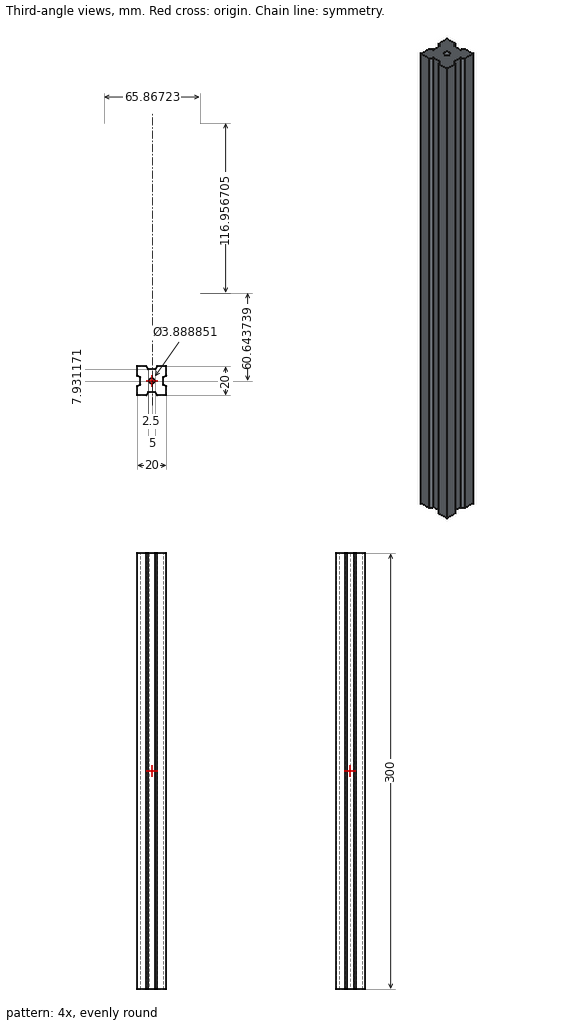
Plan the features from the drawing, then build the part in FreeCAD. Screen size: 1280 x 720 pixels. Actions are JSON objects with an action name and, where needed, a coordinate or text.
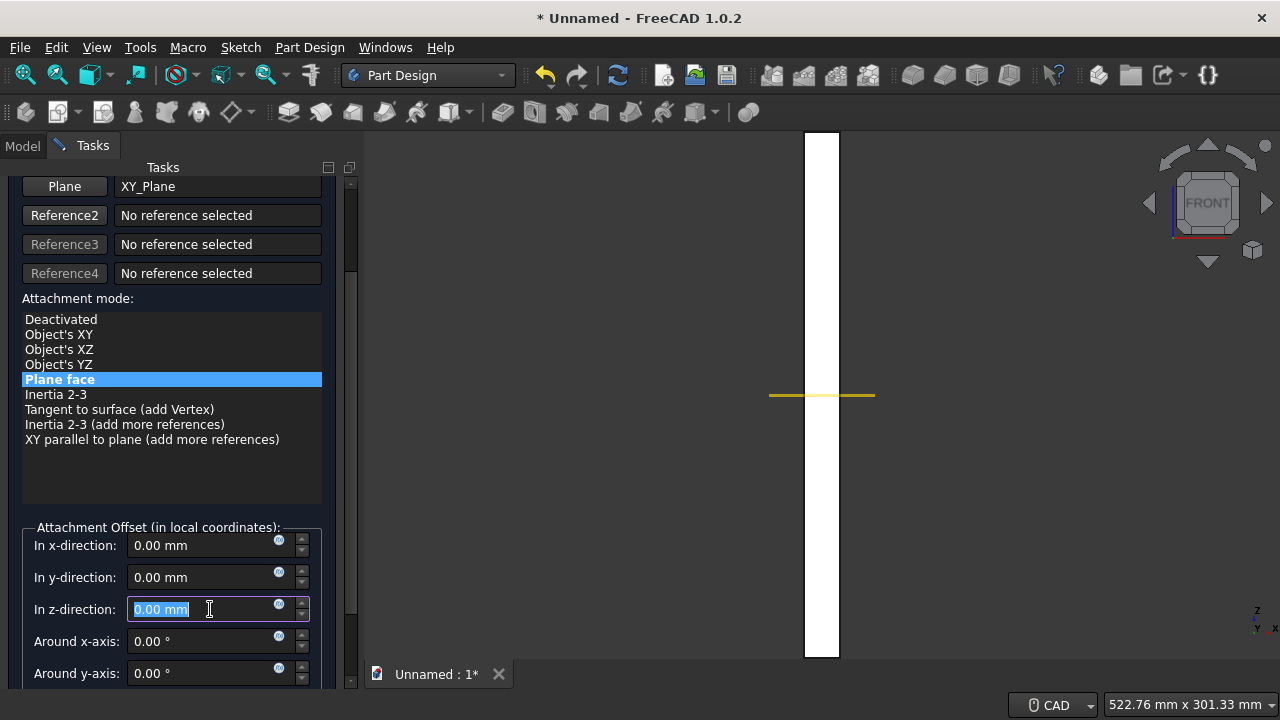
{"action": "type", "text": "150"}
{"action": "key", "text": "Tab"}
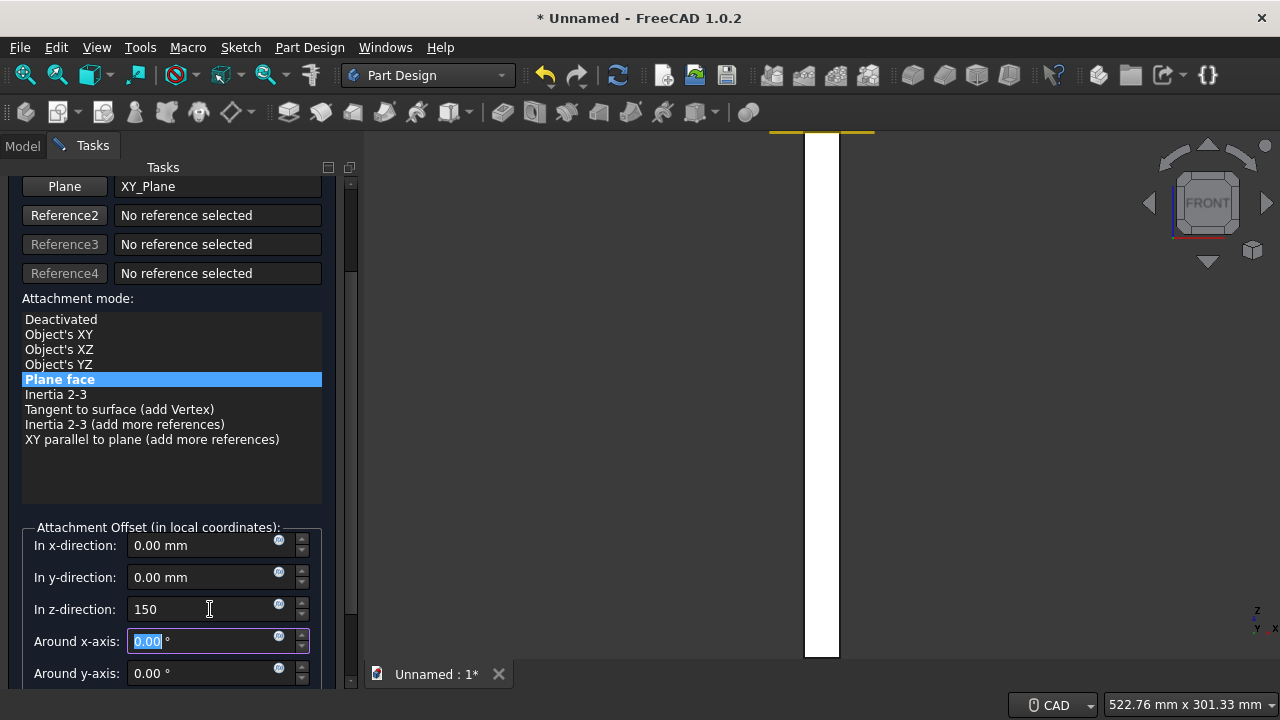
{"action": "scroll", "coordinate": [351, 432], "scroll_direction": "up", "scroll_amount": 3}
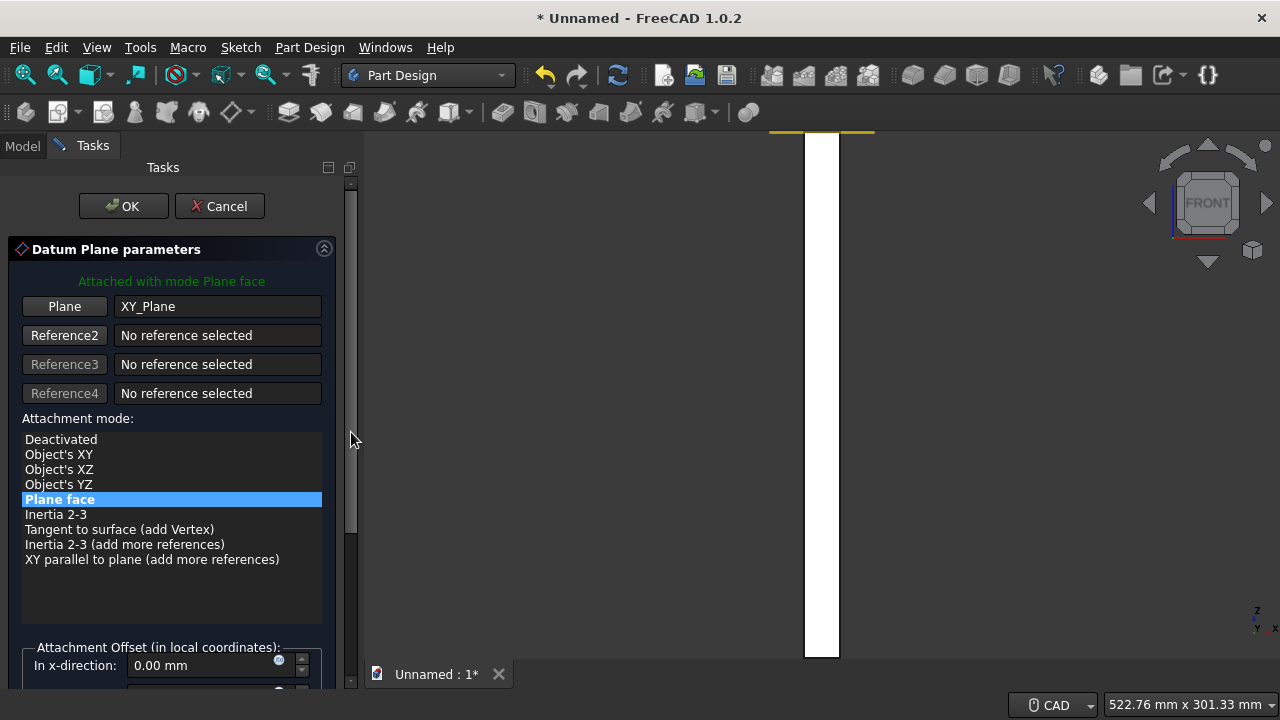
{"action": "left_click", "coordinate": [124, 206]}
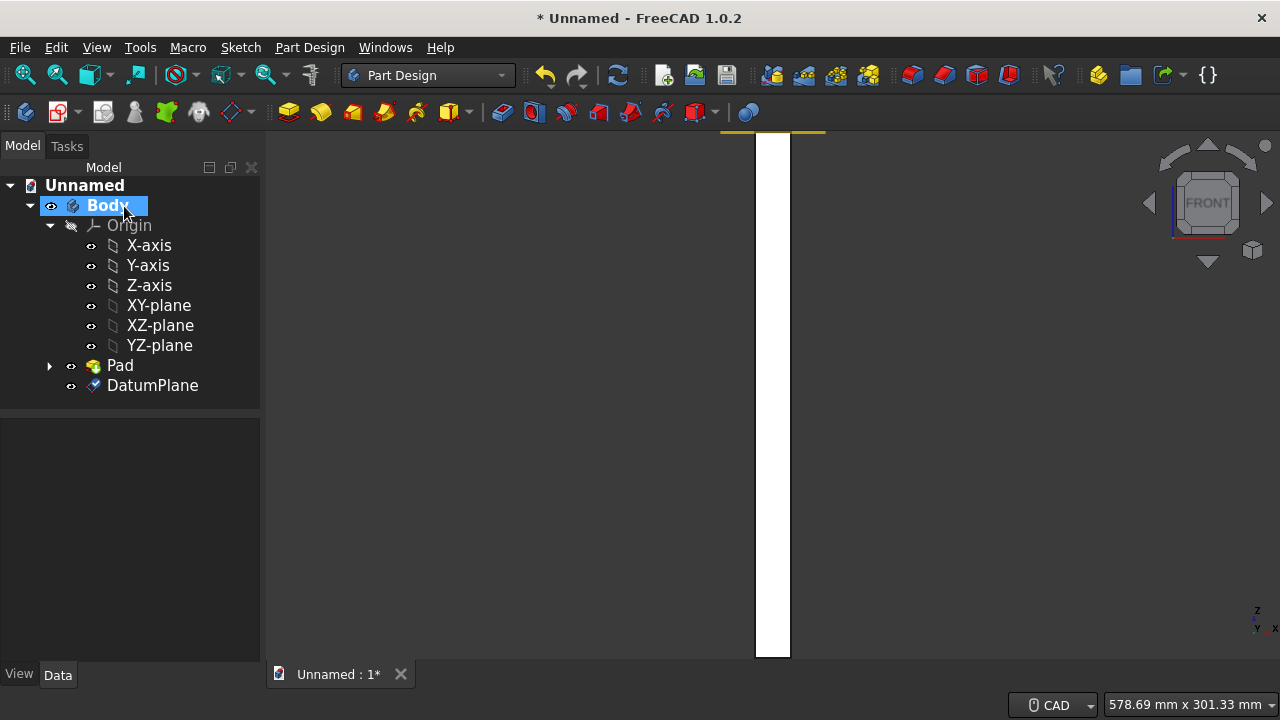
{"action": "left_click", "coordinate": [116, 386]}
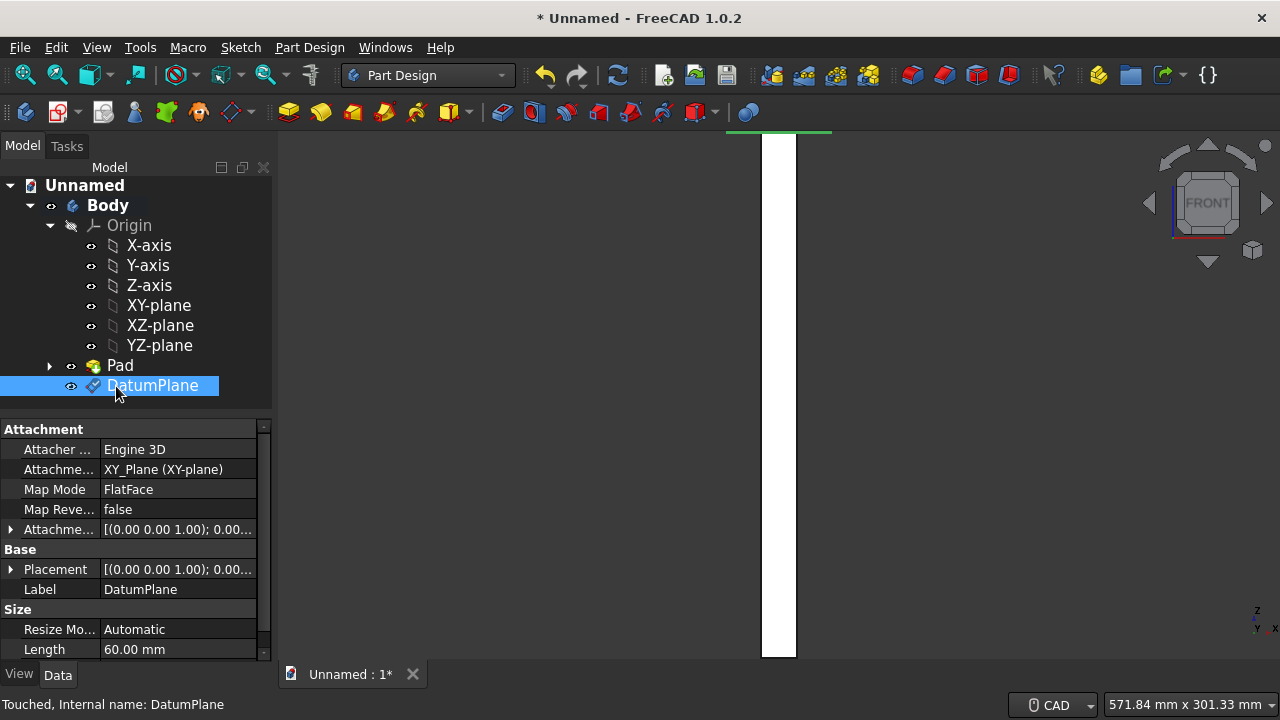
{"action": "left_click", "coordinate": [58, 112]}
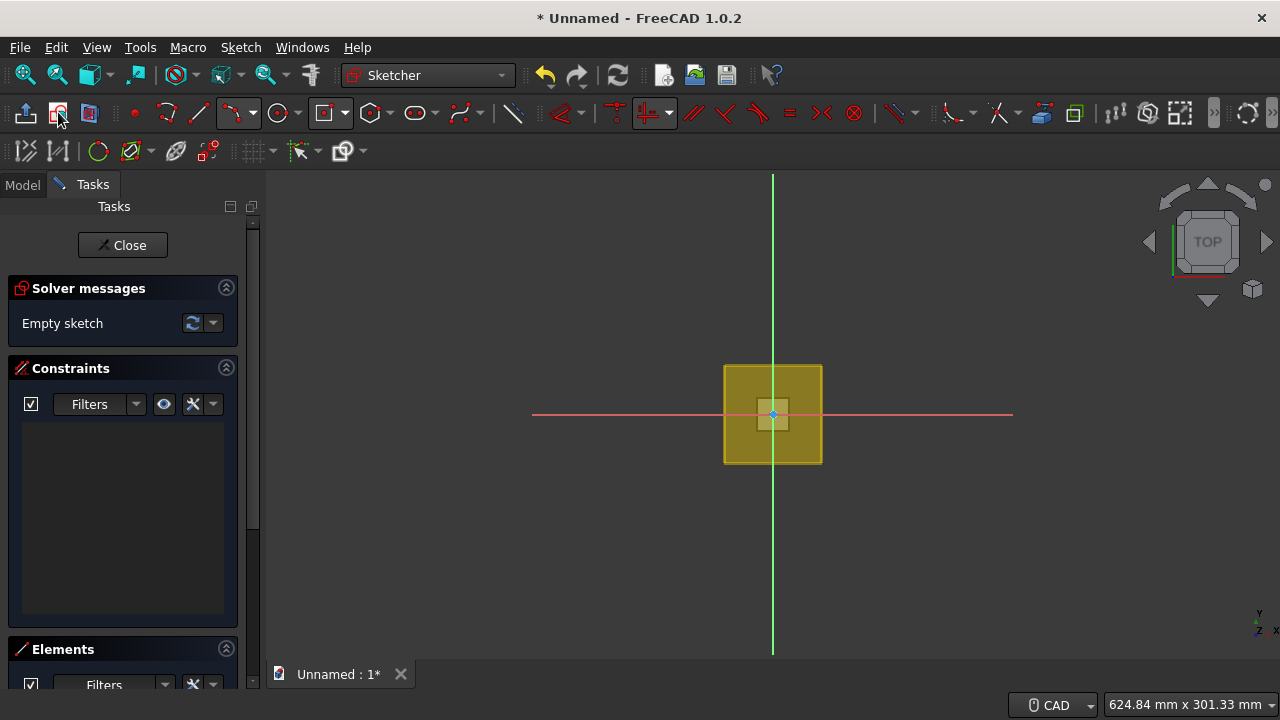
{"action": "scroll", "coordinate": [565, 631], "scroll_direction": "down", "scroll_amount": 2}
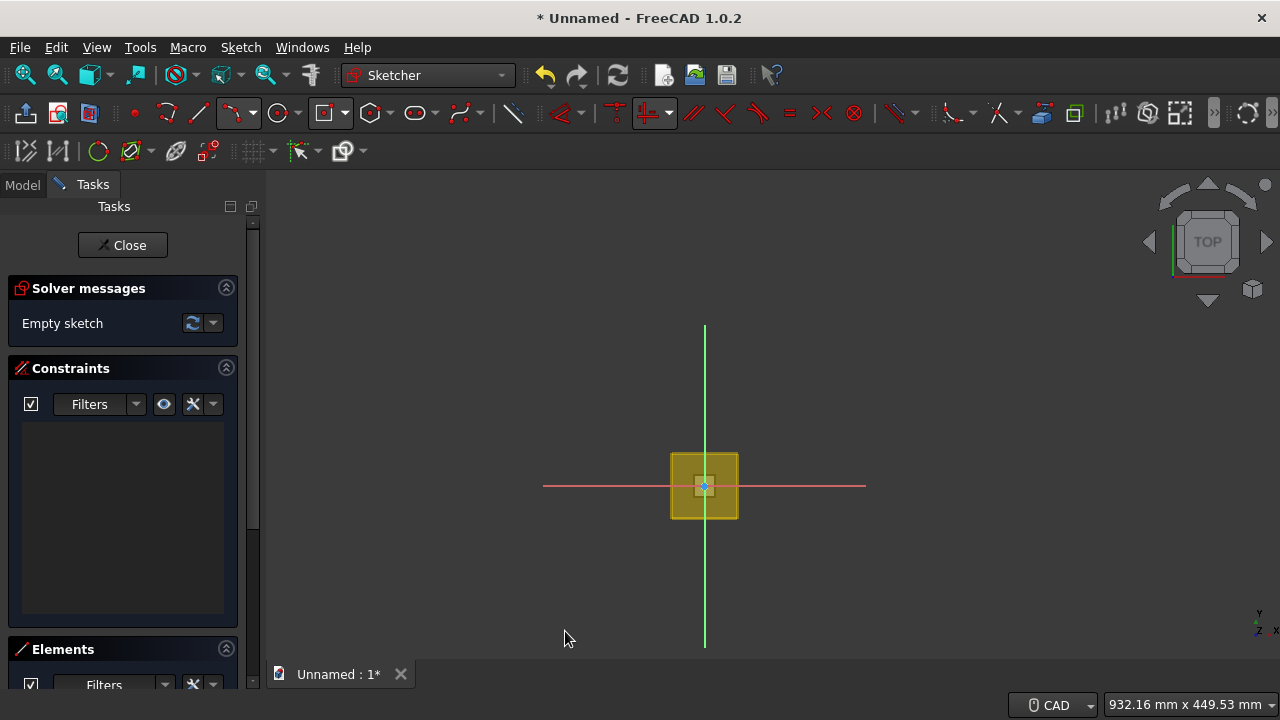
{"action": "scroll", "coordinate": [705, 339], "scroll_direction": "up", "scroll_amount": 2}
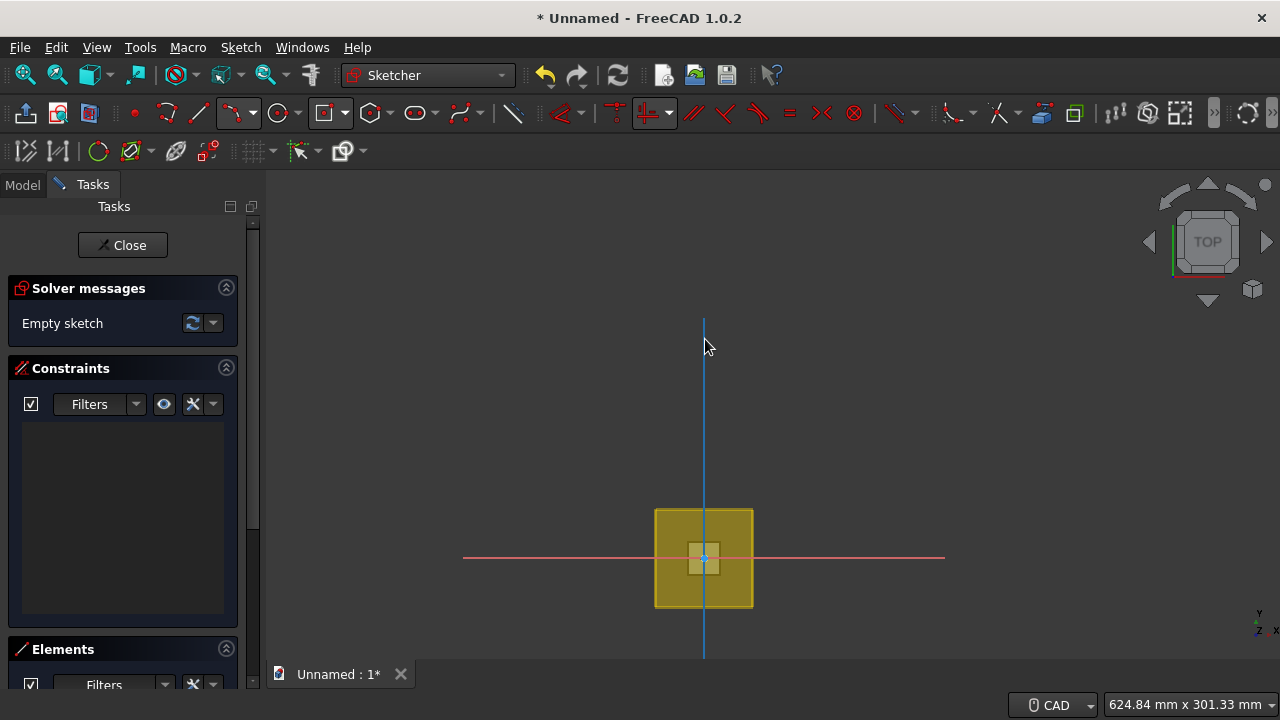
{"action": "left_click", "coordinate": [168, 114]}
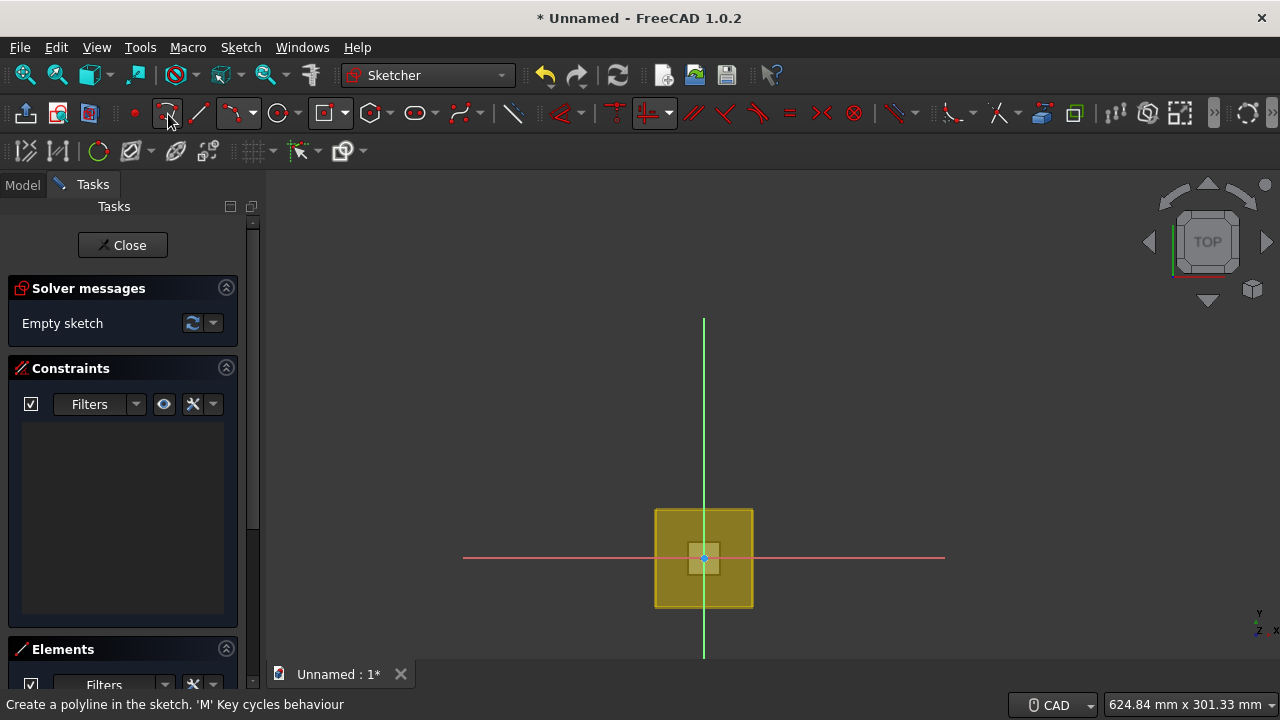
{"action": "scroll", "coordinate": [700, 546], "scroll_direction": "up", "scroll_amount": 7}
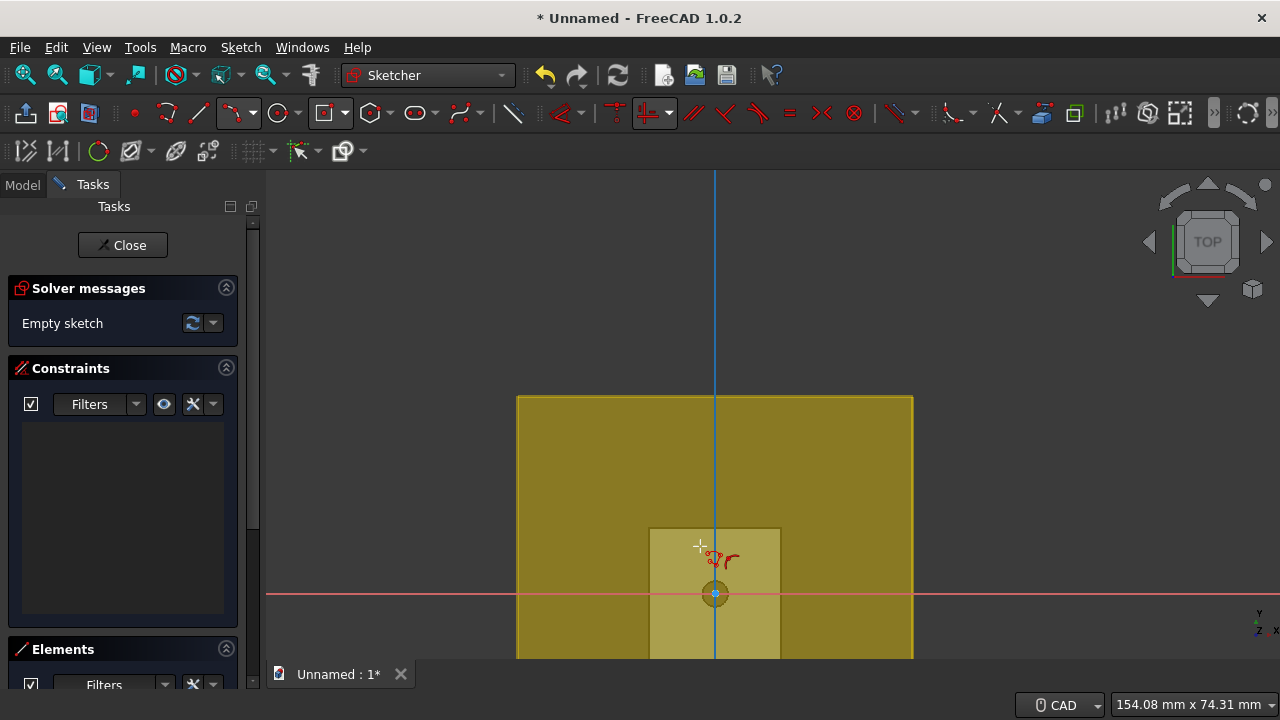
{"action": "left_click", "coordinate": [699, 542]}
{"action": "left_click", "coordinate": [732, 542]}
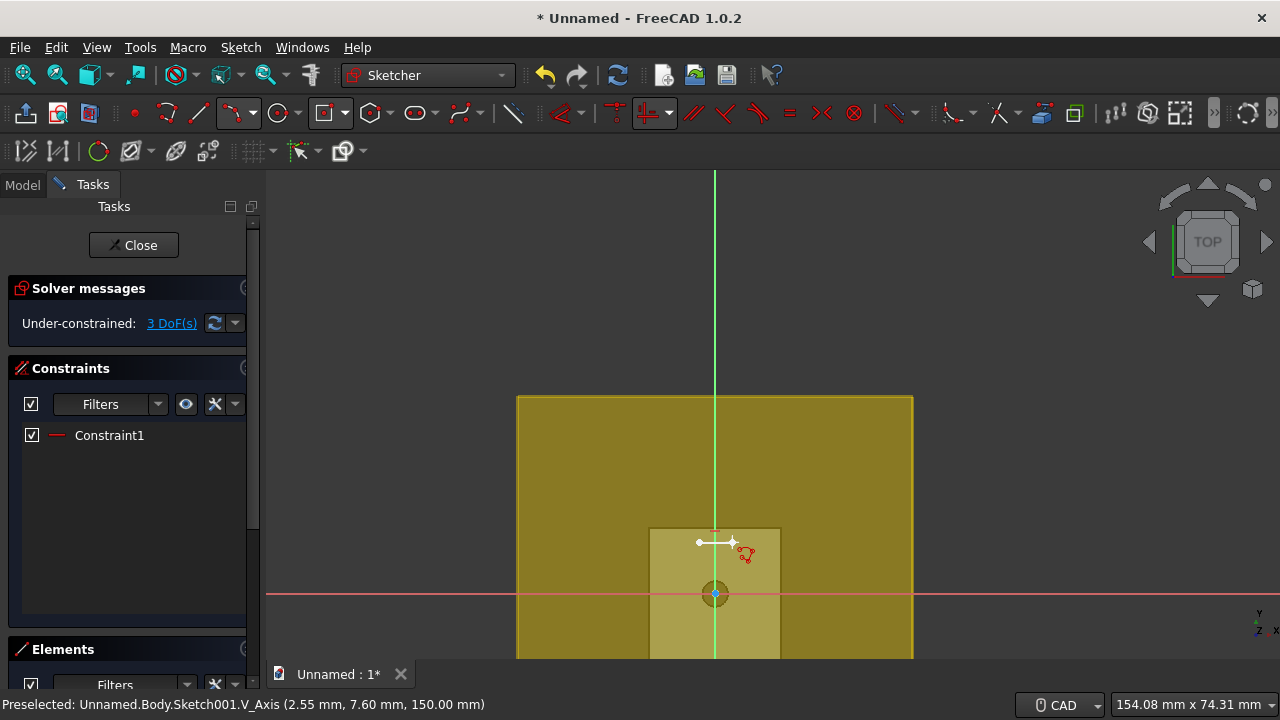
{"action": "scroll", "coordinate": [701, 547], "scroll_direction": "down", "scroll_amount": 7}